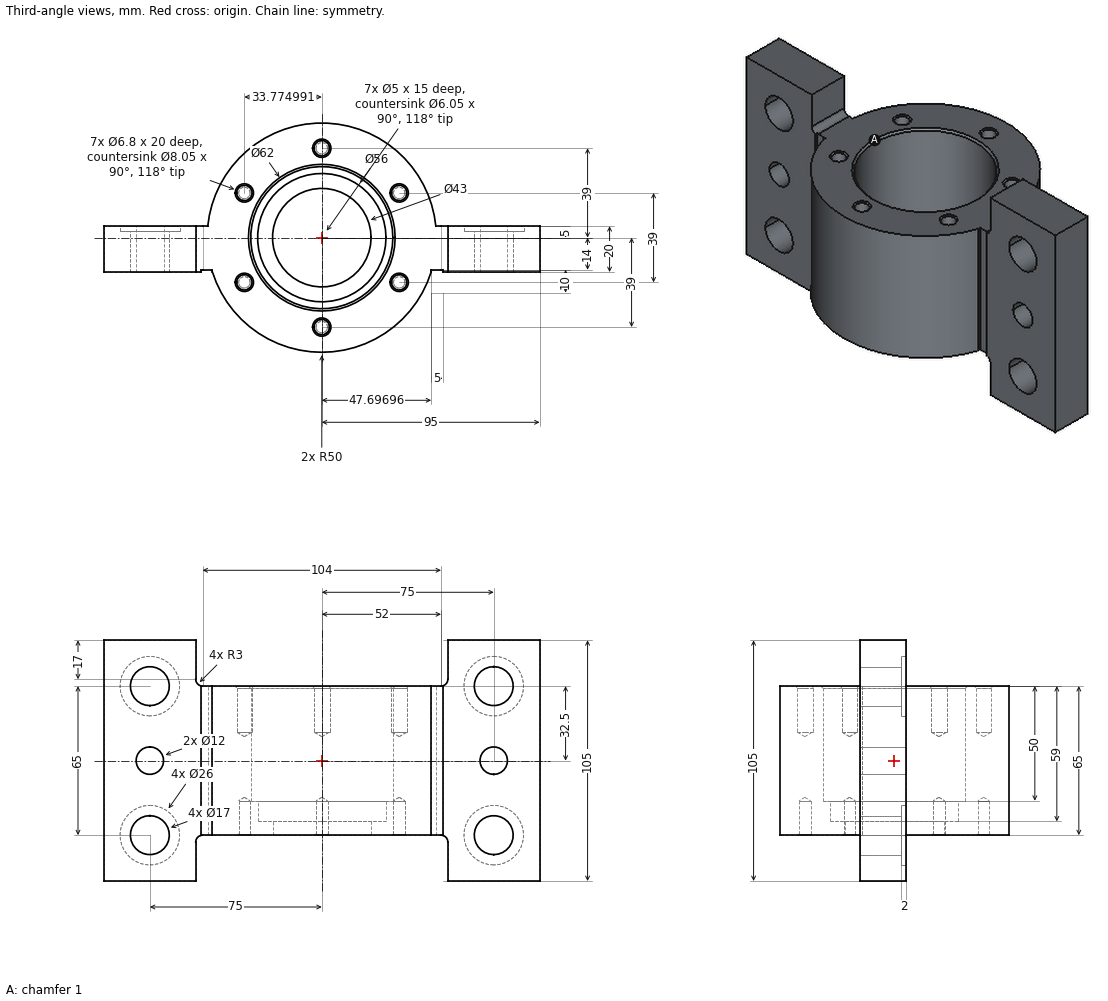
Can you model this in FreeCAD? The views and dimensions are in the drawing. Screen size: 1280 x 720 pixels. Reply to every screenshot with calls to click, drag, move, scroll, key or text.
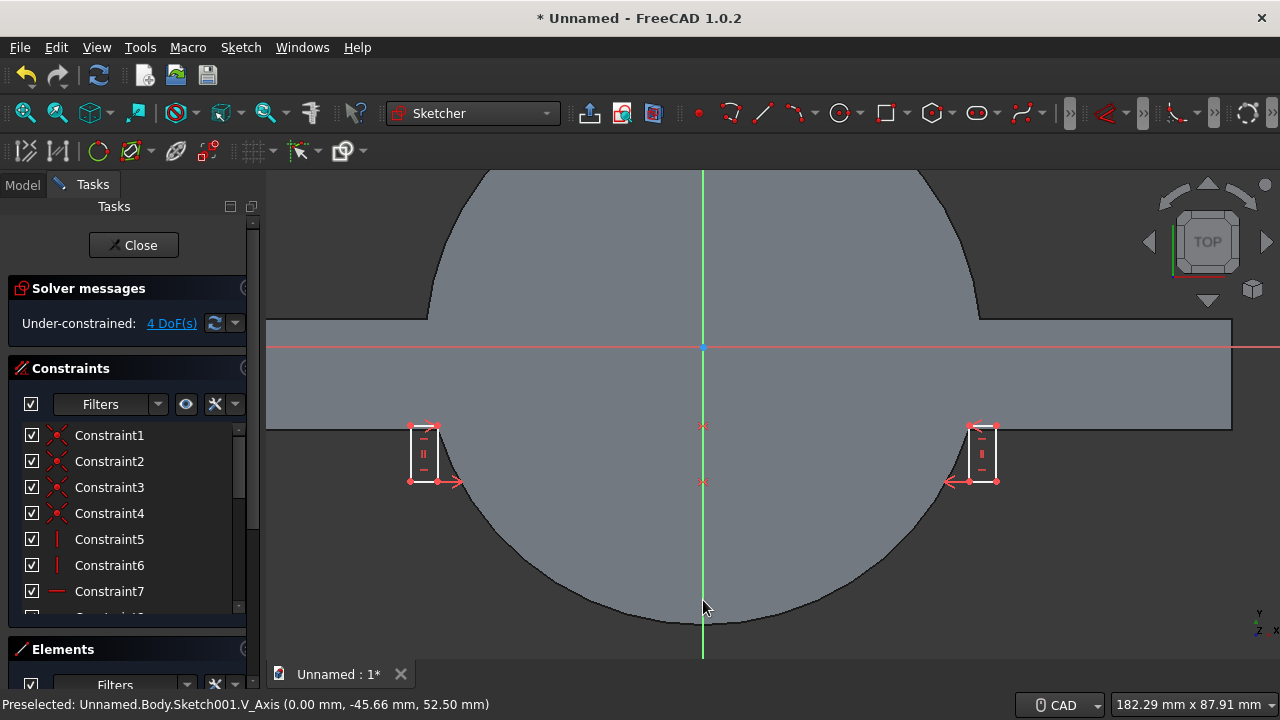
click(1106, 114)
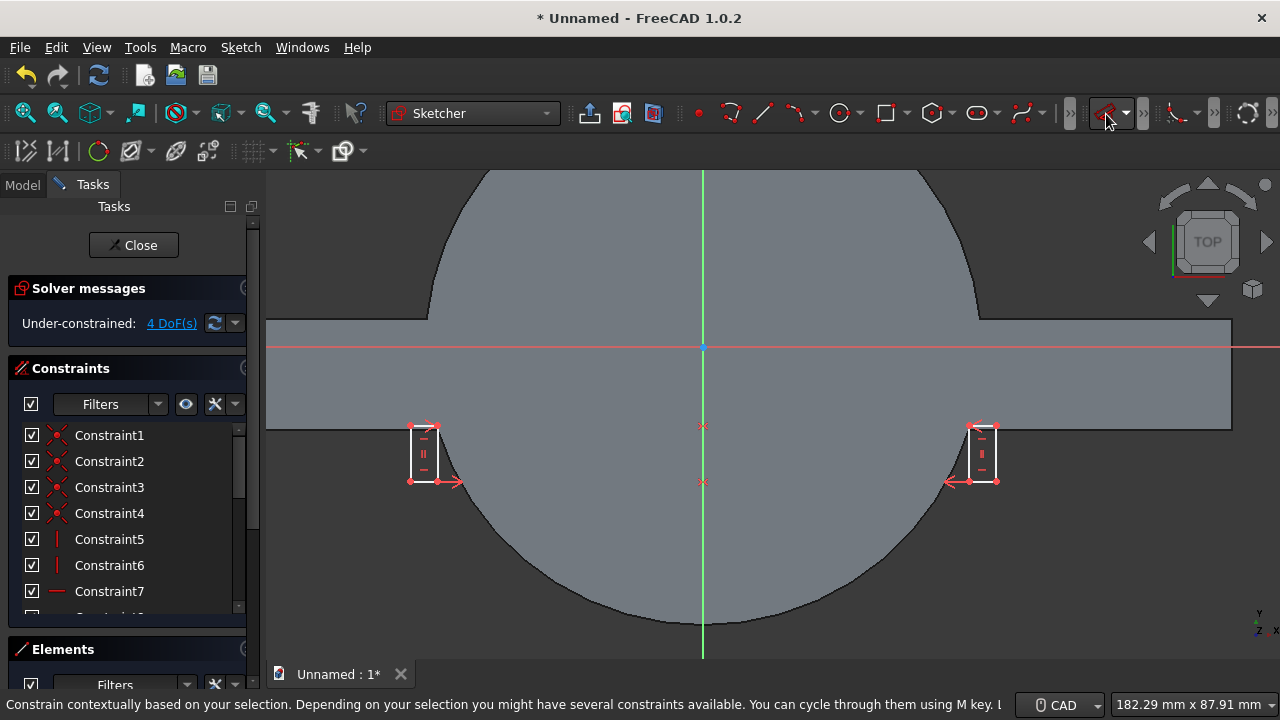
scroll(980, 482, up, 2)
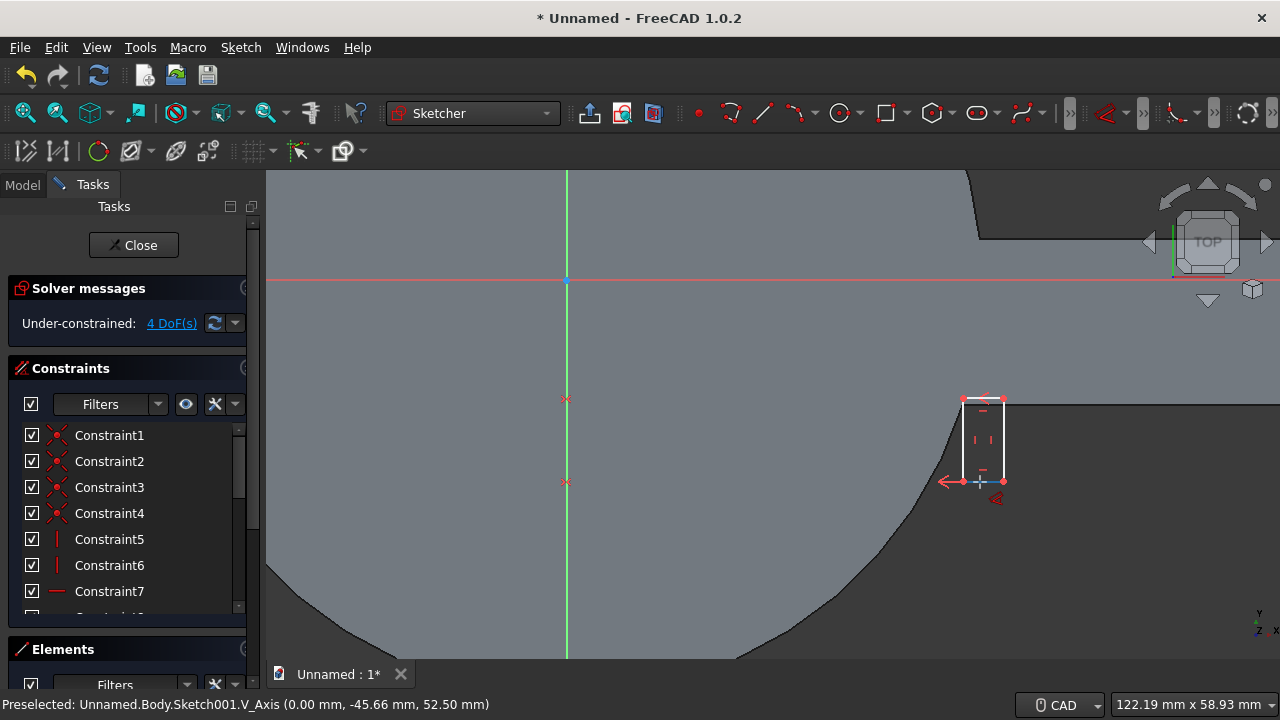
click(979, 482)
click(983, 516)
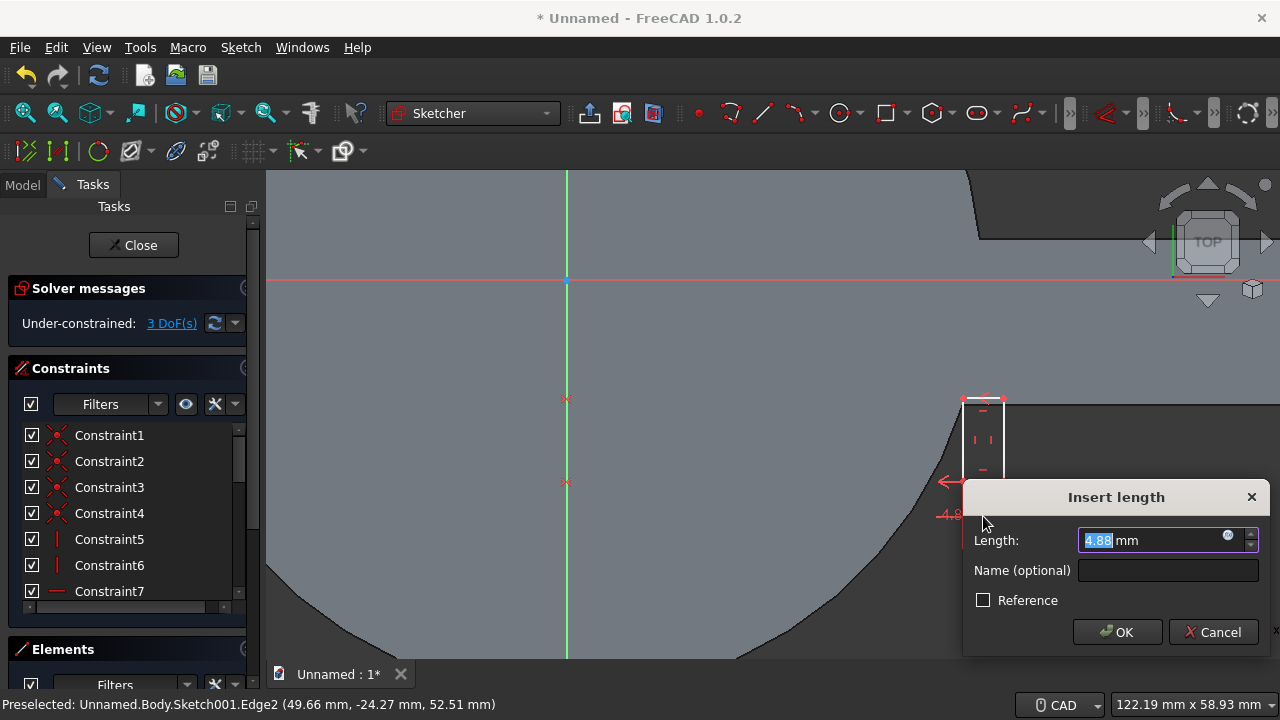
text(5)
key(Return)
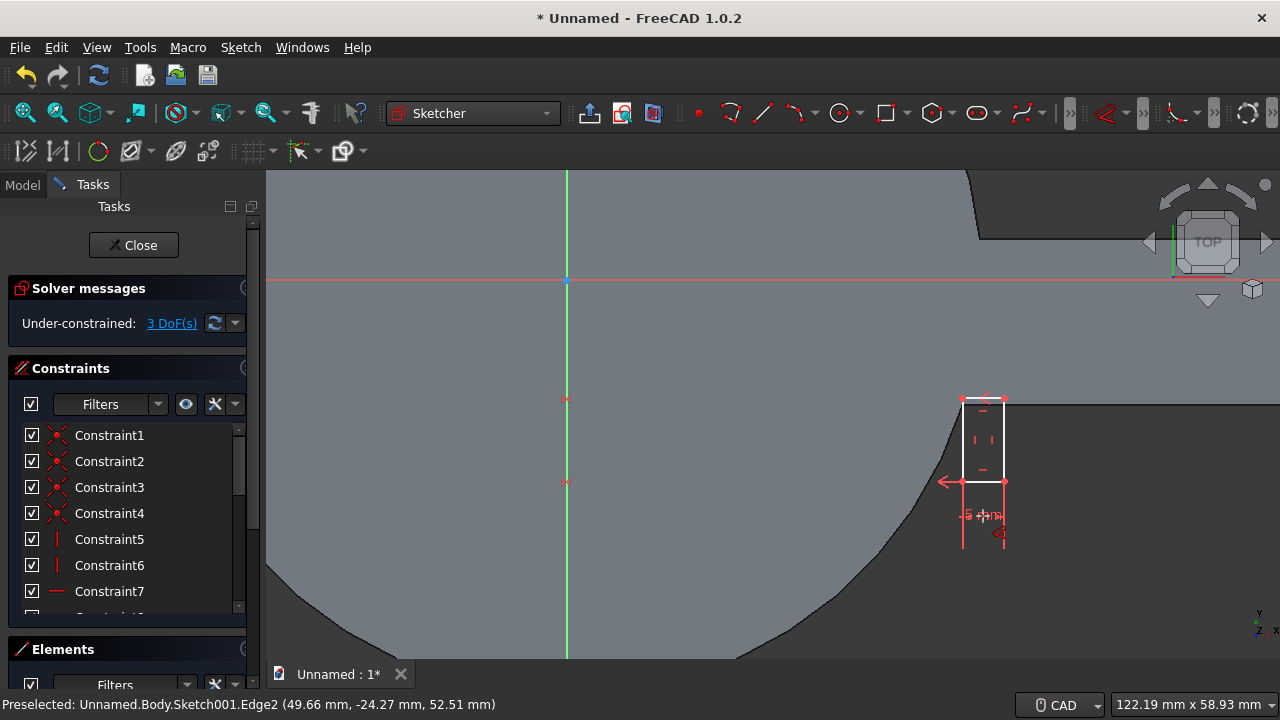
click(963, 423)
click(929, 440)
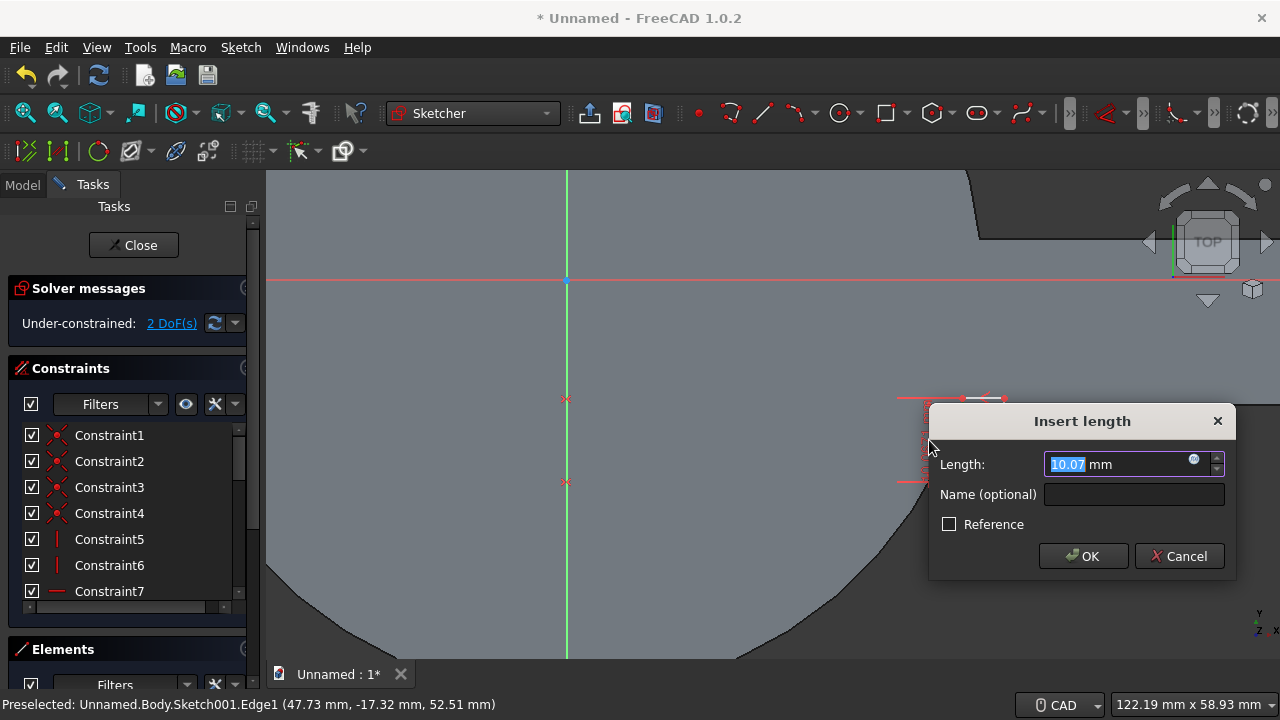
text(10)
key(Return)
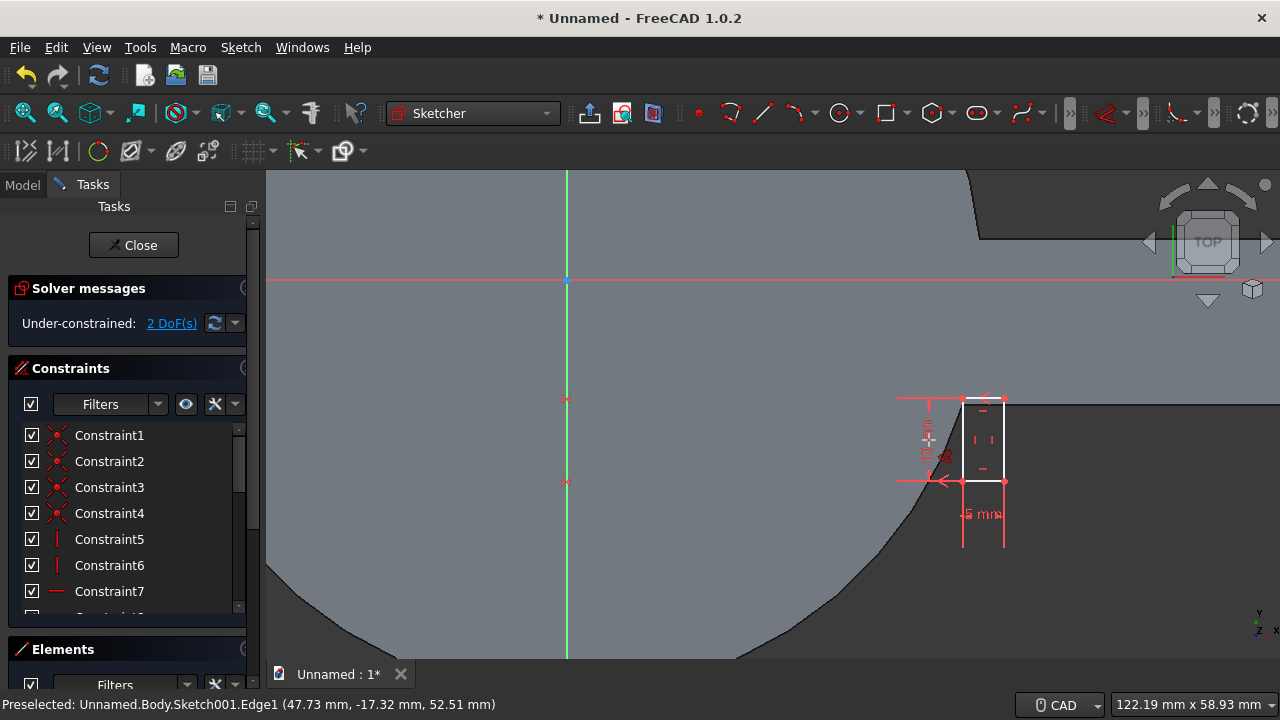
click(963, 398)
click(997, 339)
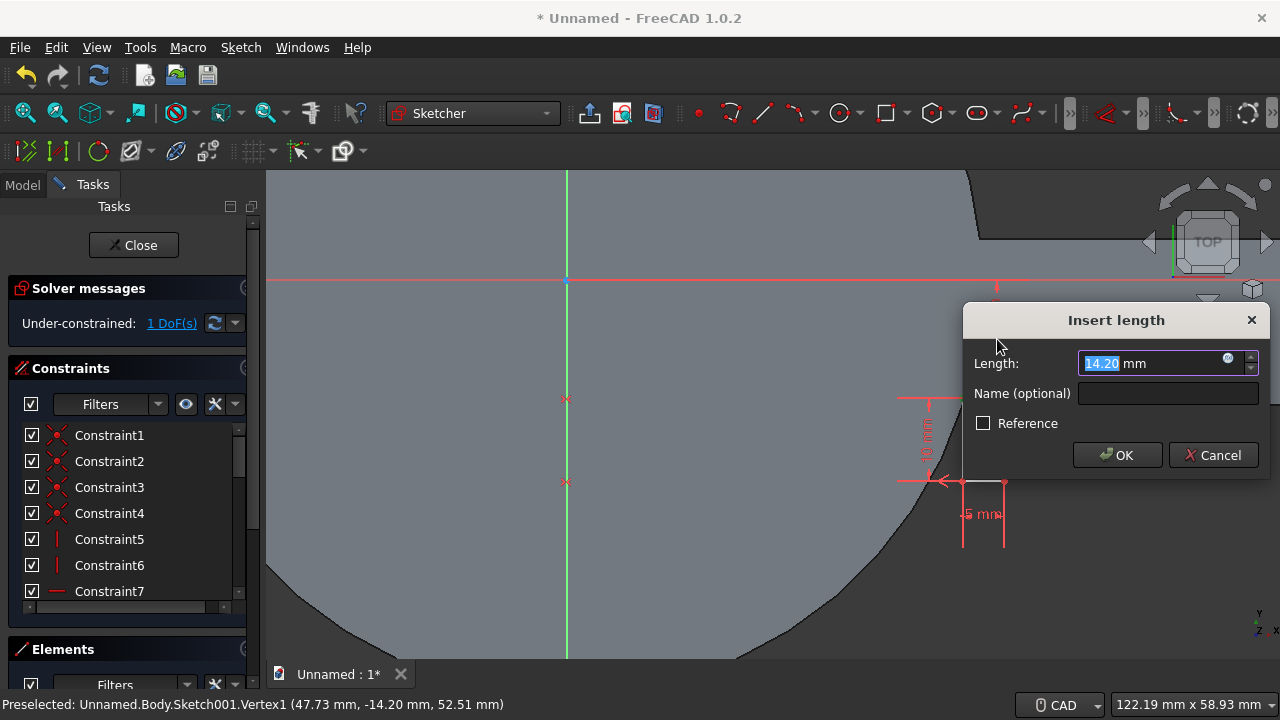
text(14)
key(Return)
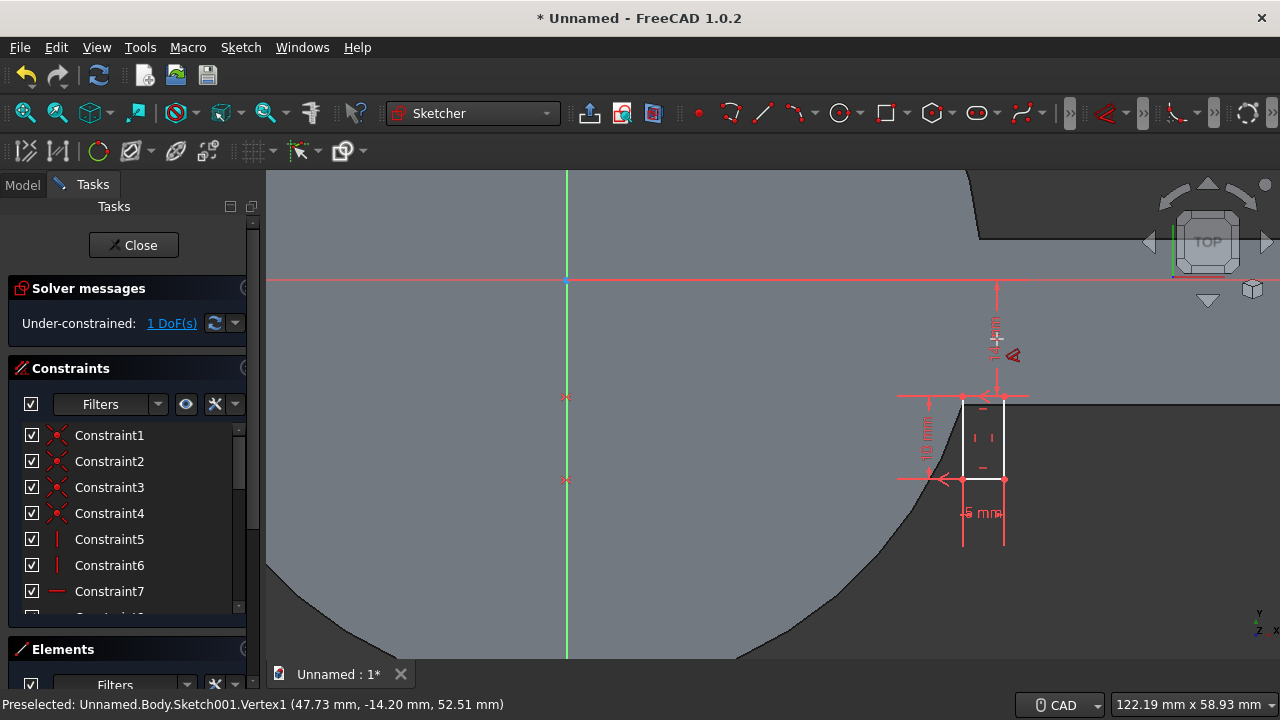
click(963, 396)
click(765, 246)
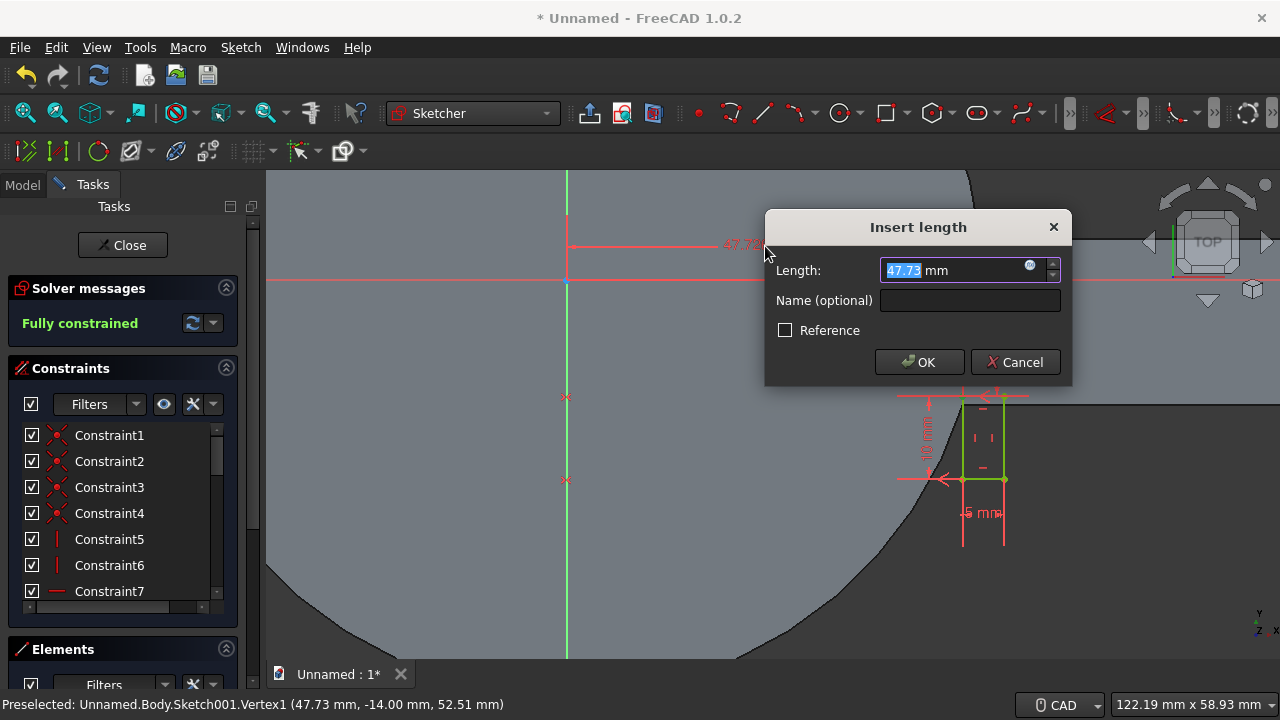
text(47.69696)
key(Return)
key(Escape)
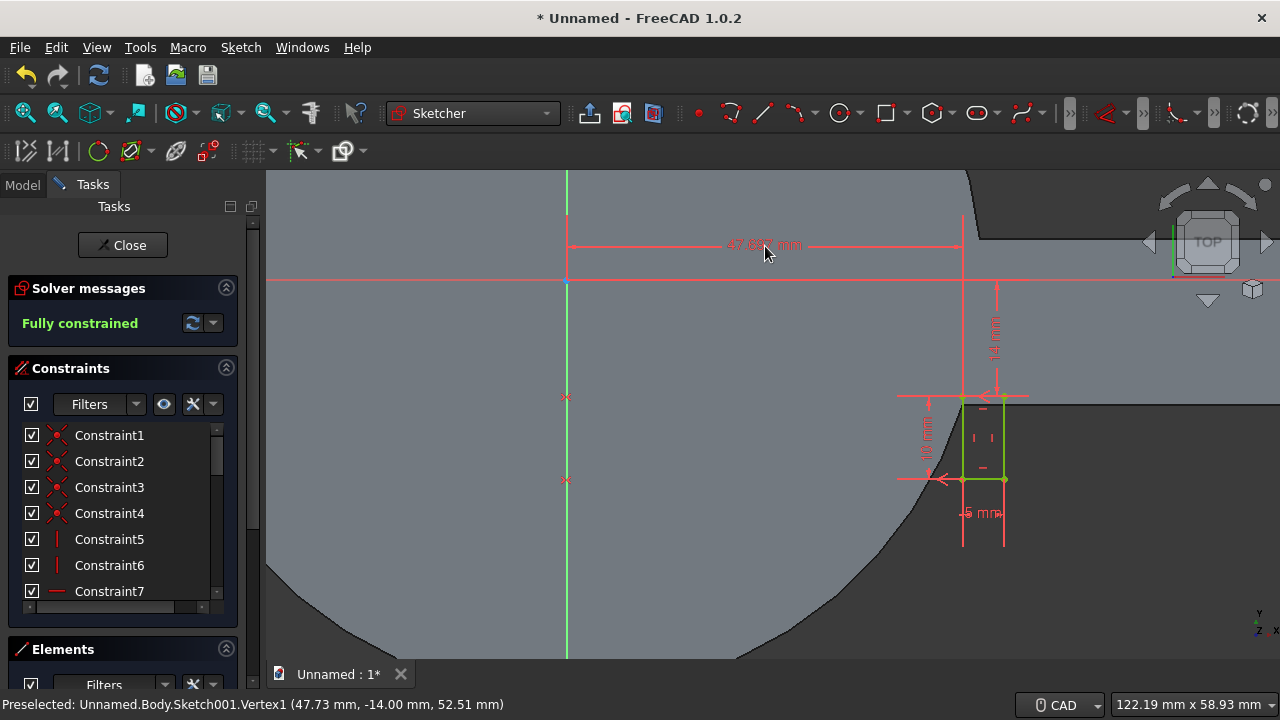
click(123, 245)